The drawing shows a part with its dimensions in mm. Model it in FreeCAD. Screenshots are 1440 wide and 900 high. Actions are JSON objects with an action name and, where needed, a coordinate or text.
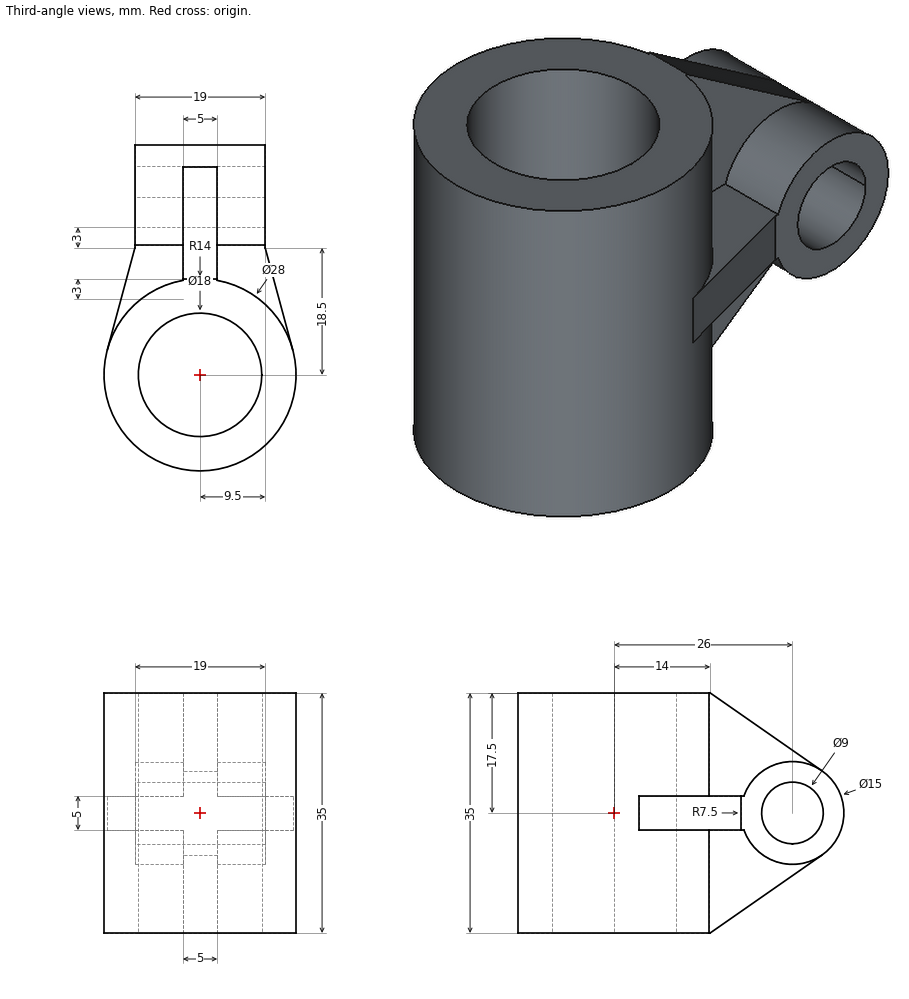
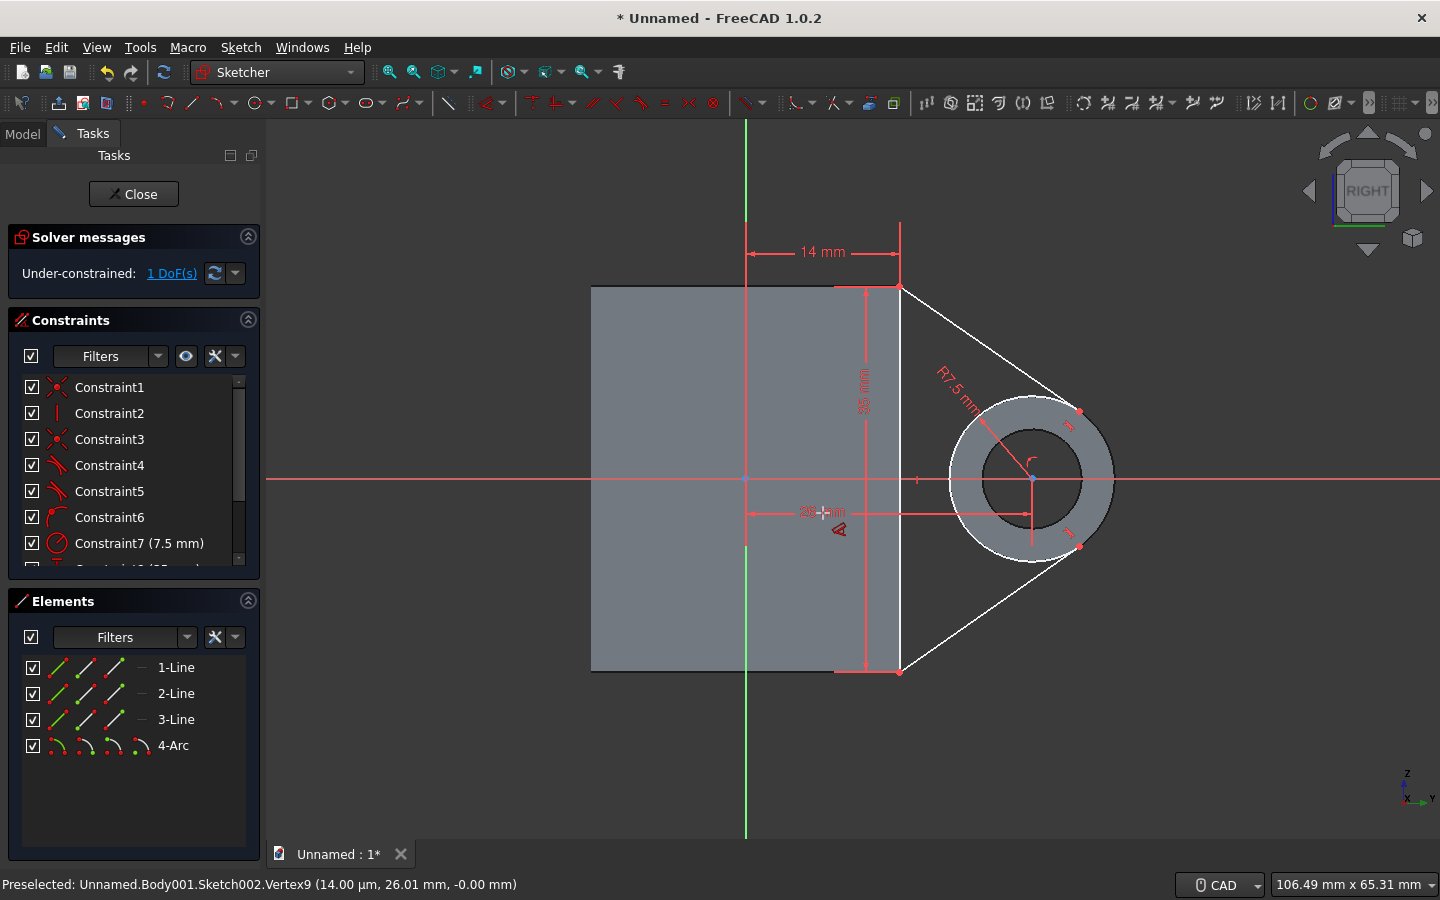
{"action": "left_click", "coordinate": [900, 287]}
{"action": "left_click", "coordinate": [712, 383]}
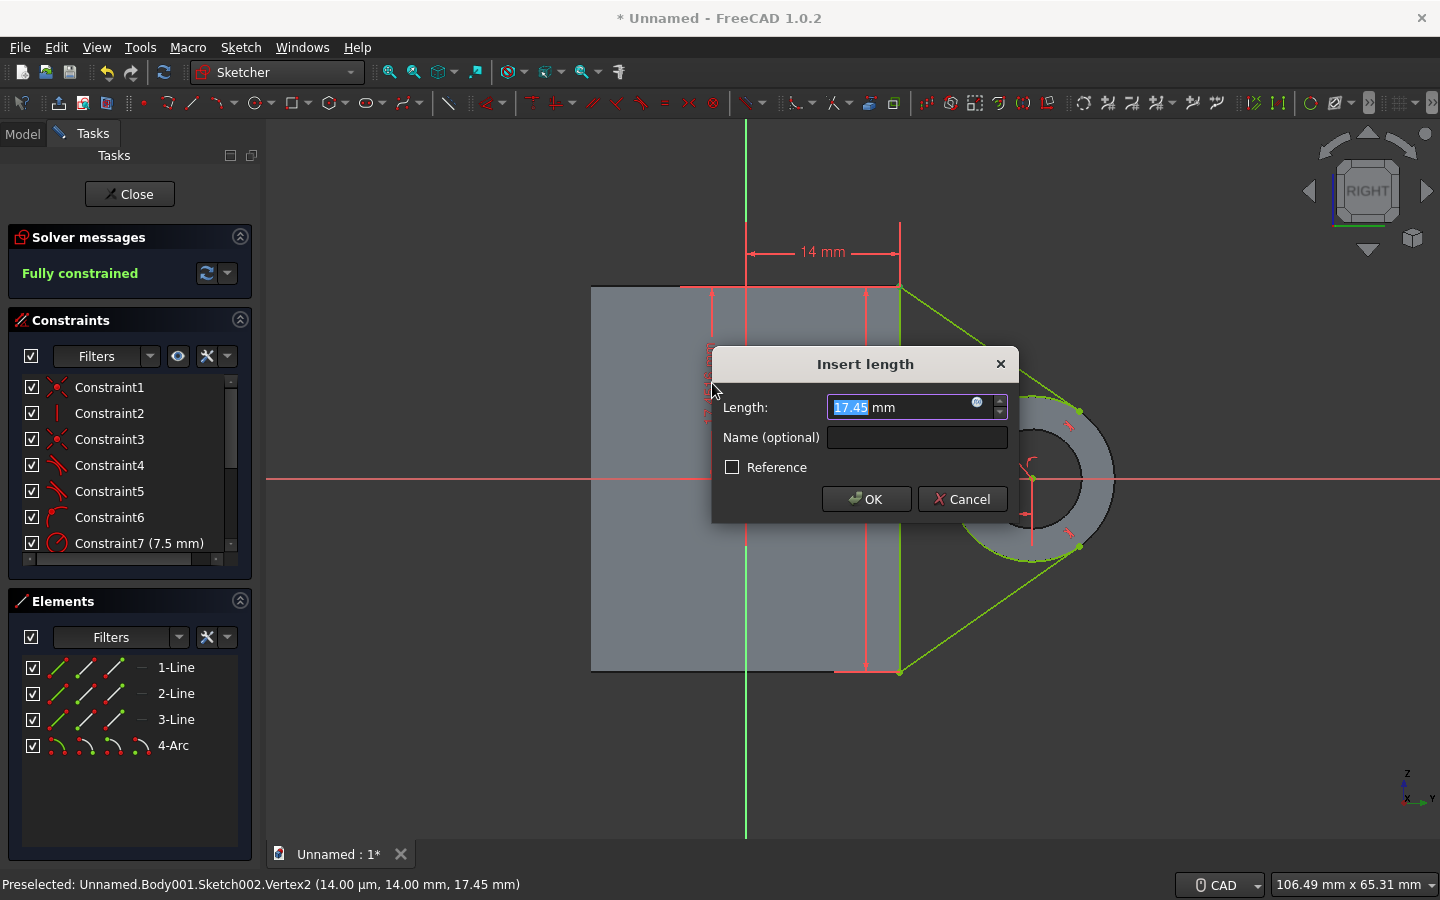
{"action": "type", "text": "17.5"}
{"action": "key", "text": "Return"}
{"action": "key", "text": "Escape"}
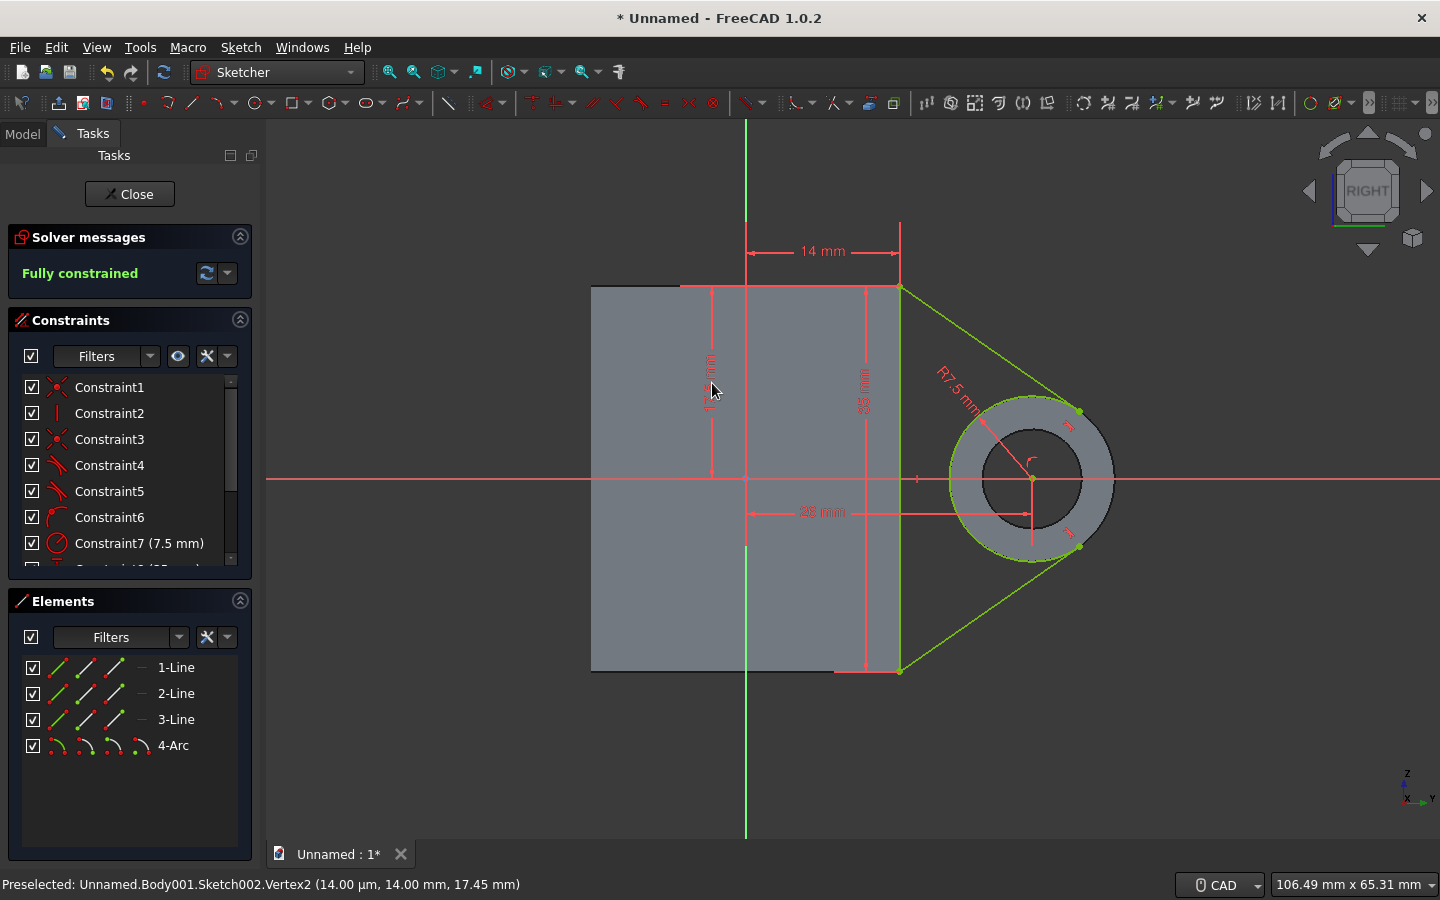
{"action": "left_click", "coordinate": [130, 194]}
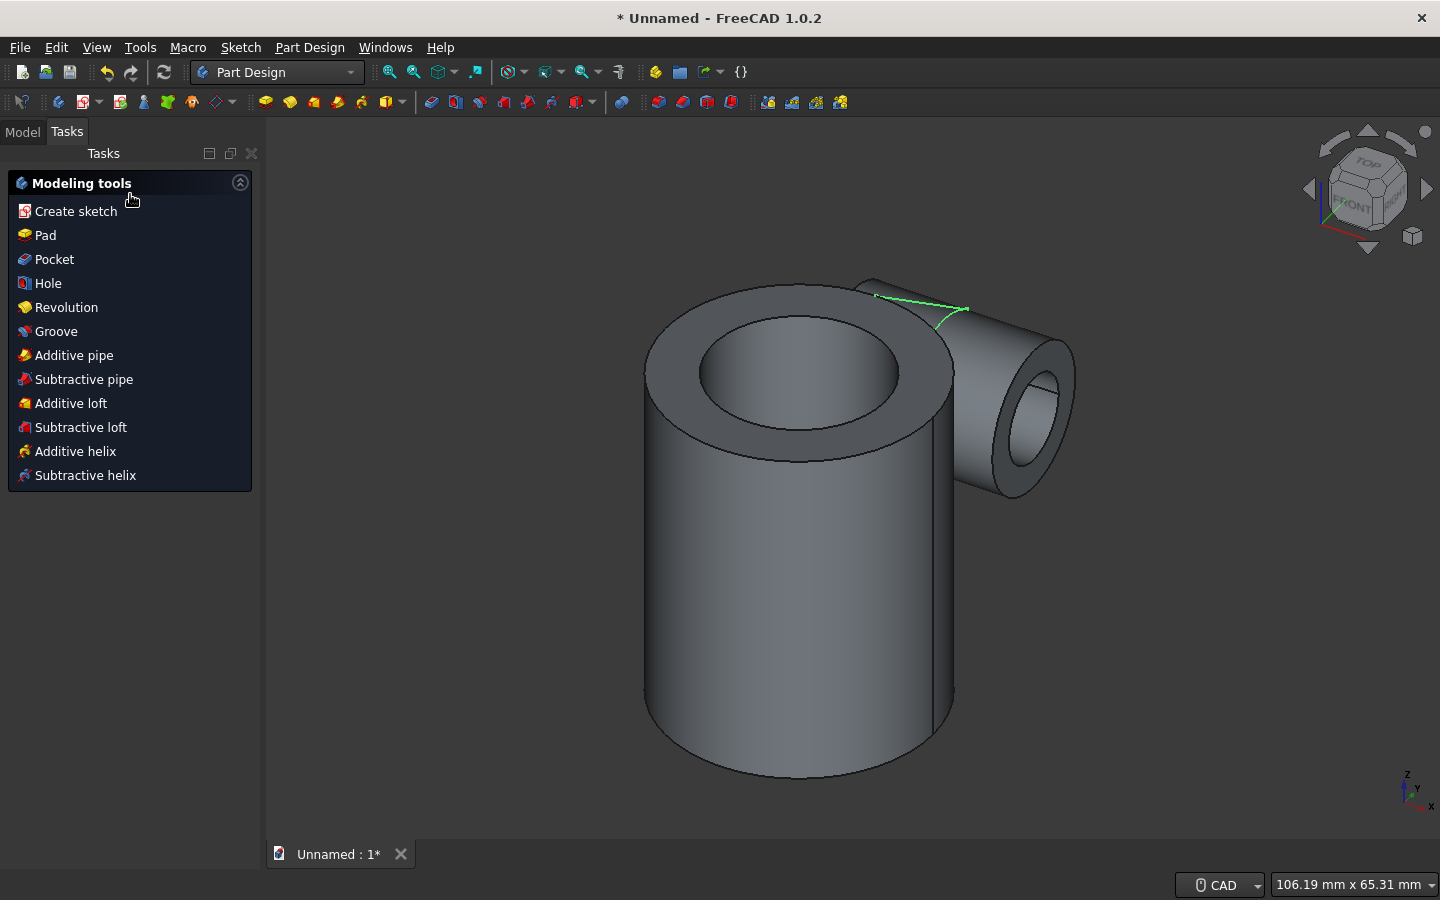
{"action": "left_click", "coordinate": [266, 102]}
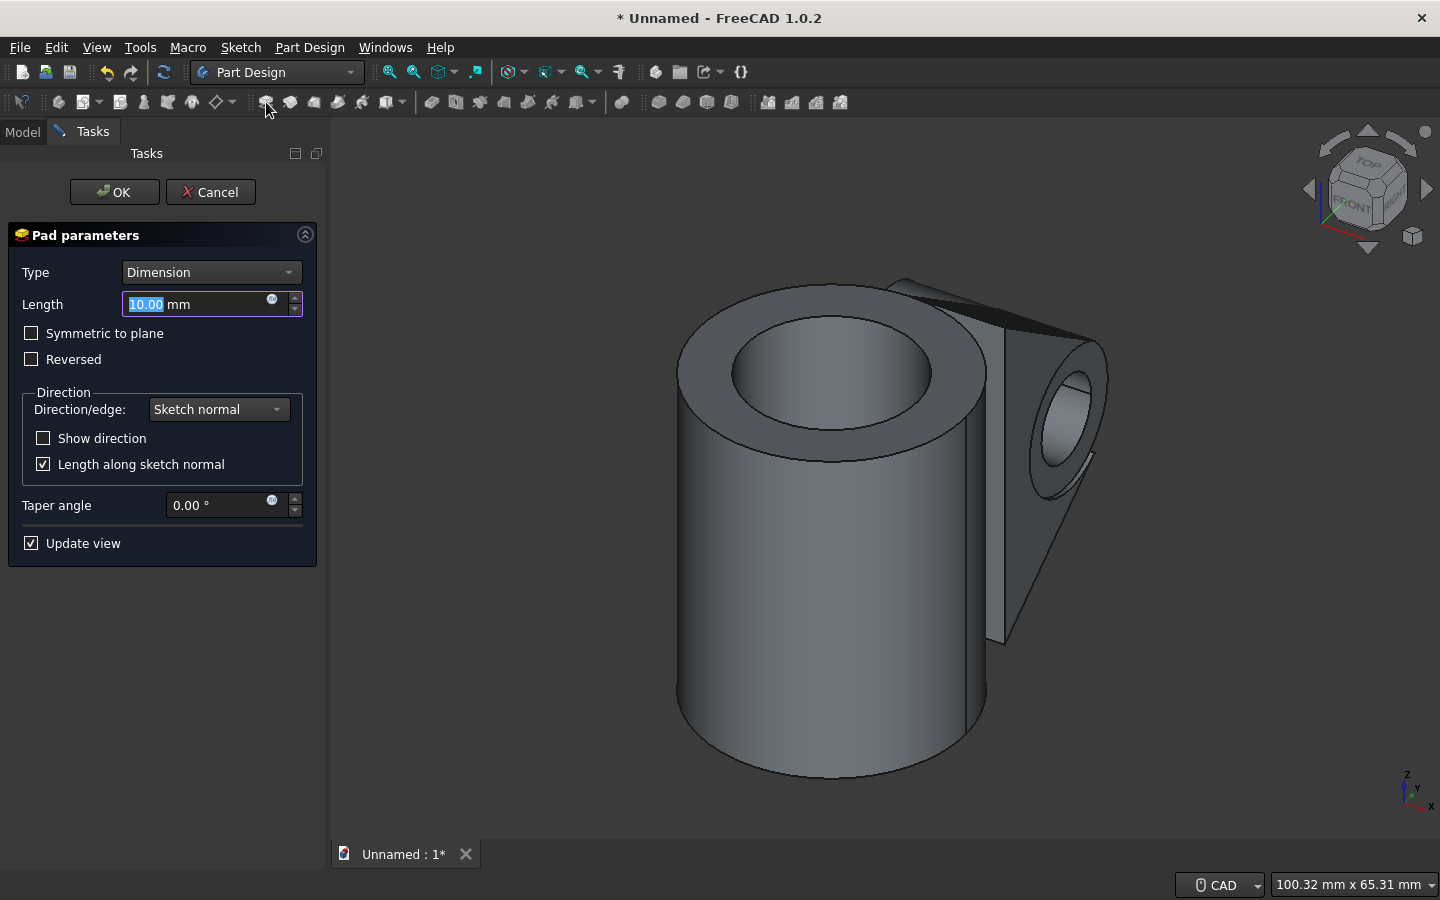
{"action": "type", "text": "5"}
{"action": "key", "text": "Tab"}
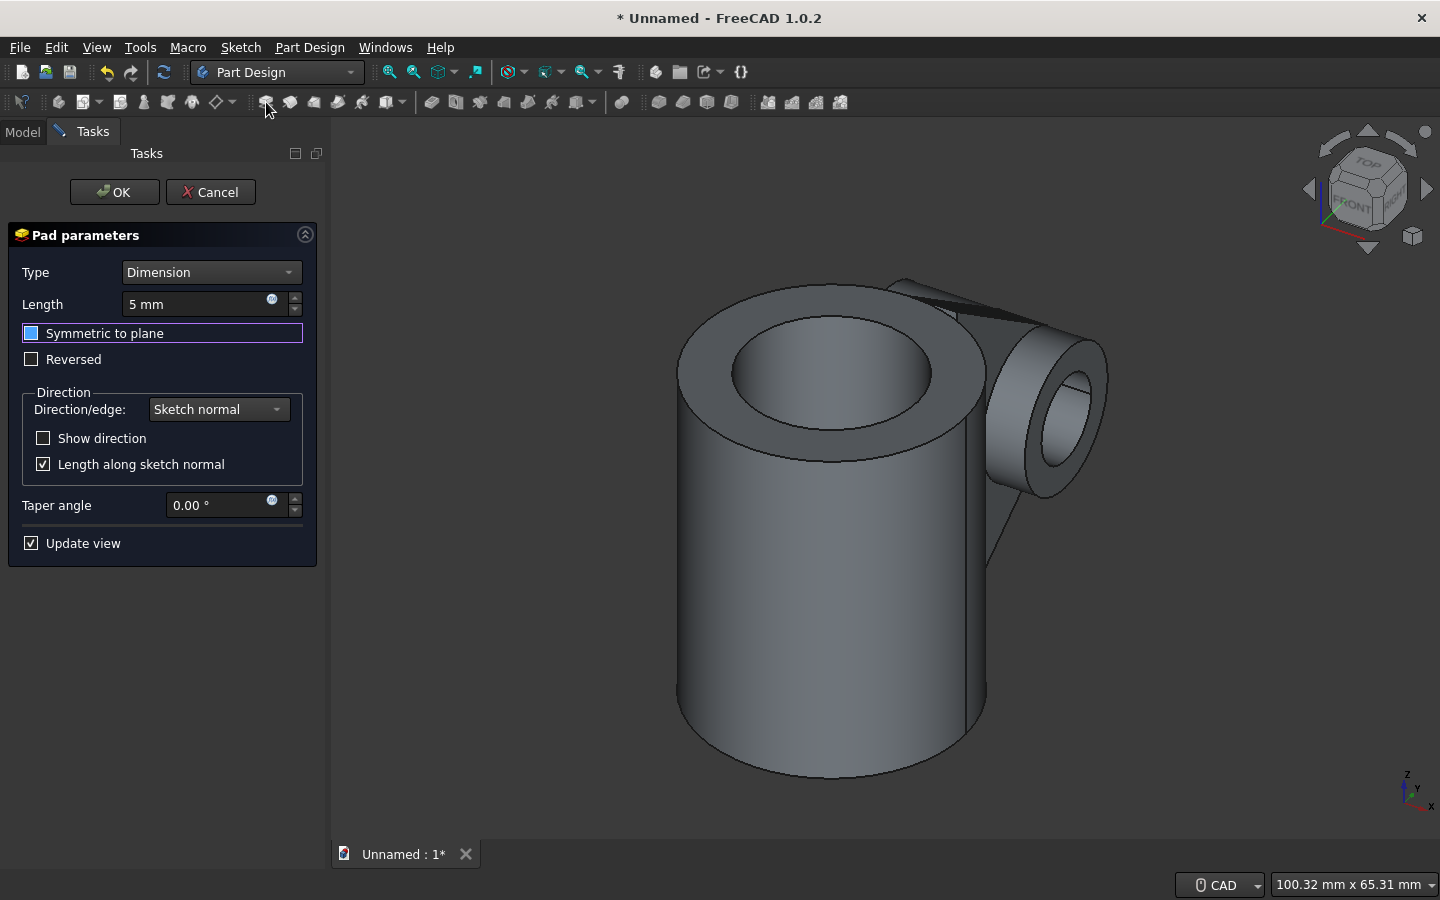
{"action": "left_click", "coordinate": [30, 333]}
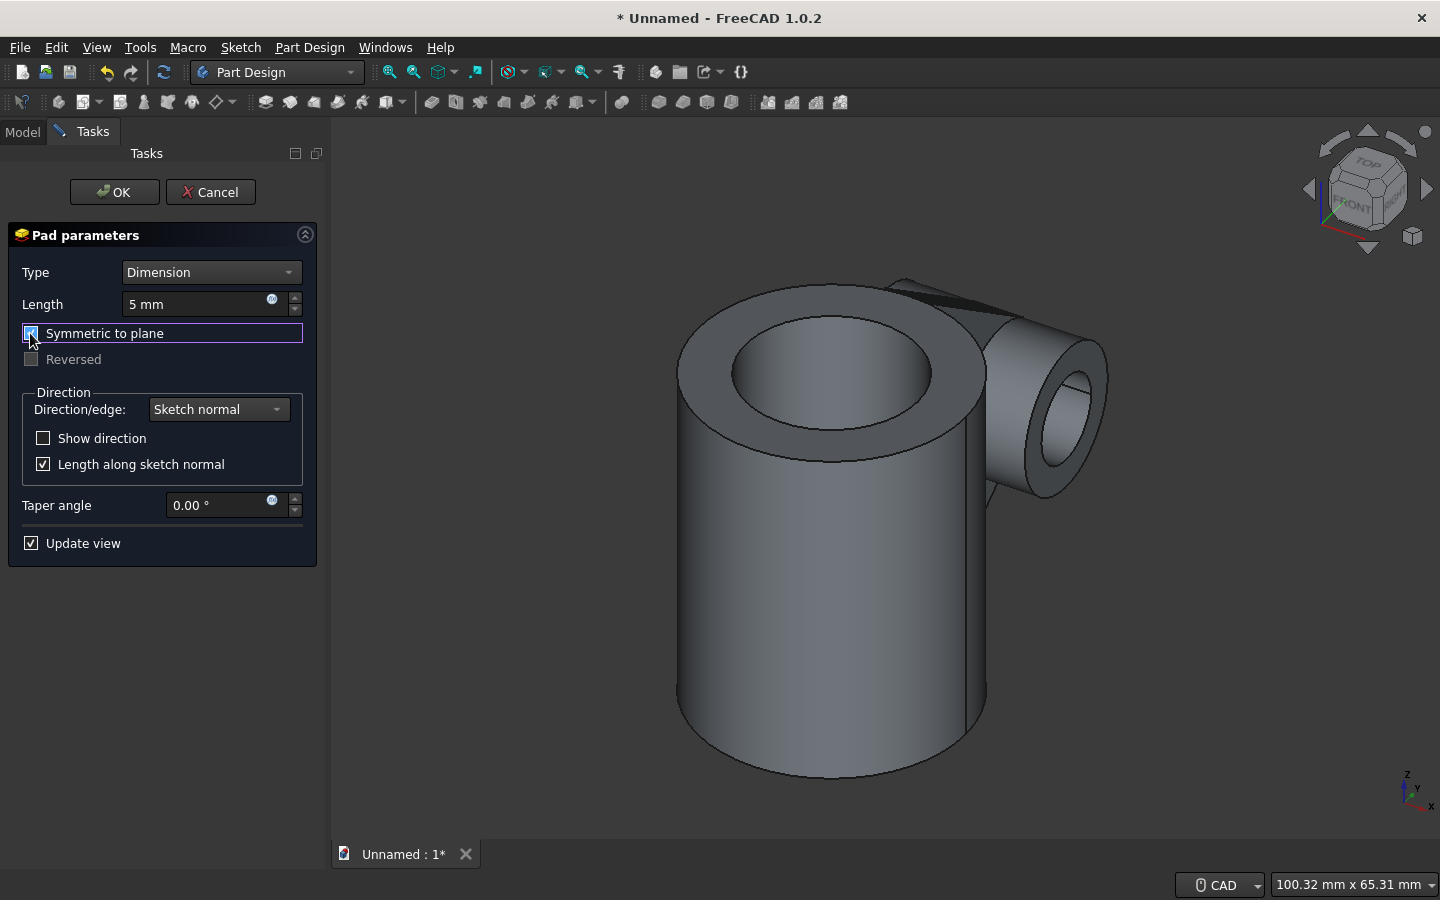
{"action": "left_click", "coordinate": [115, 192]}